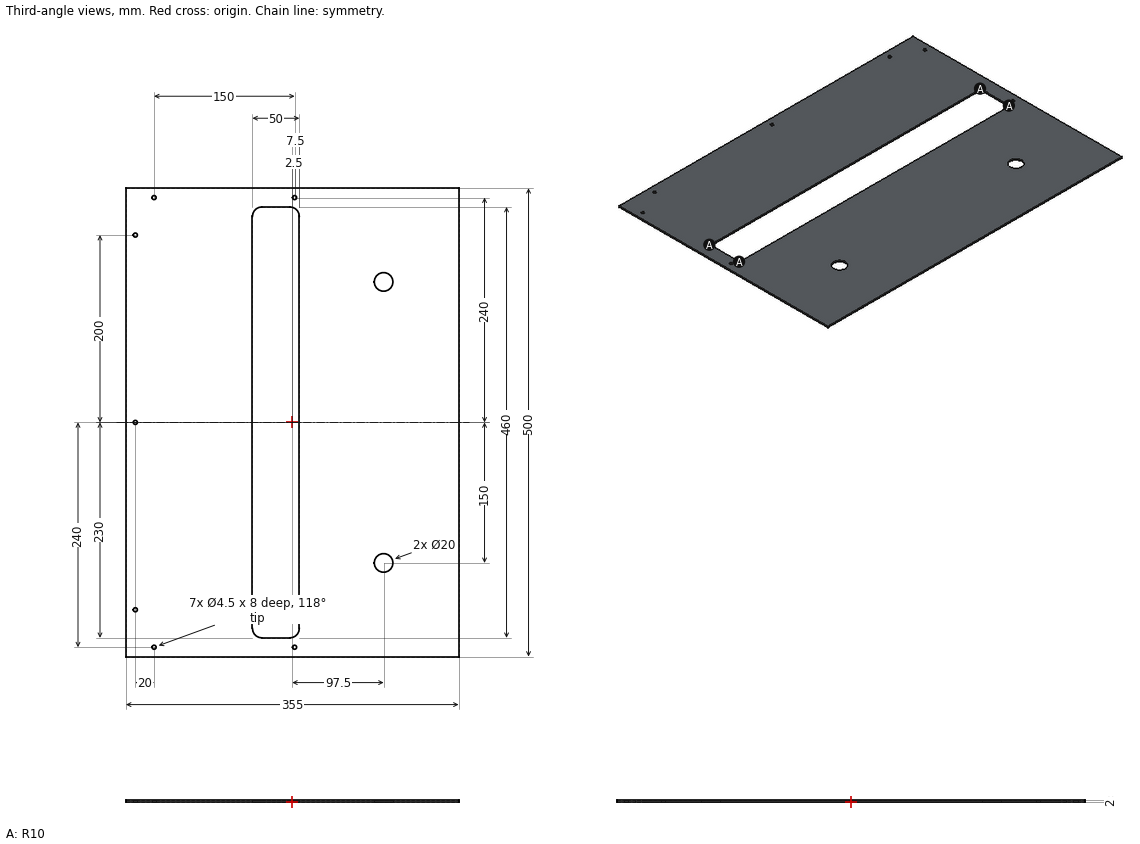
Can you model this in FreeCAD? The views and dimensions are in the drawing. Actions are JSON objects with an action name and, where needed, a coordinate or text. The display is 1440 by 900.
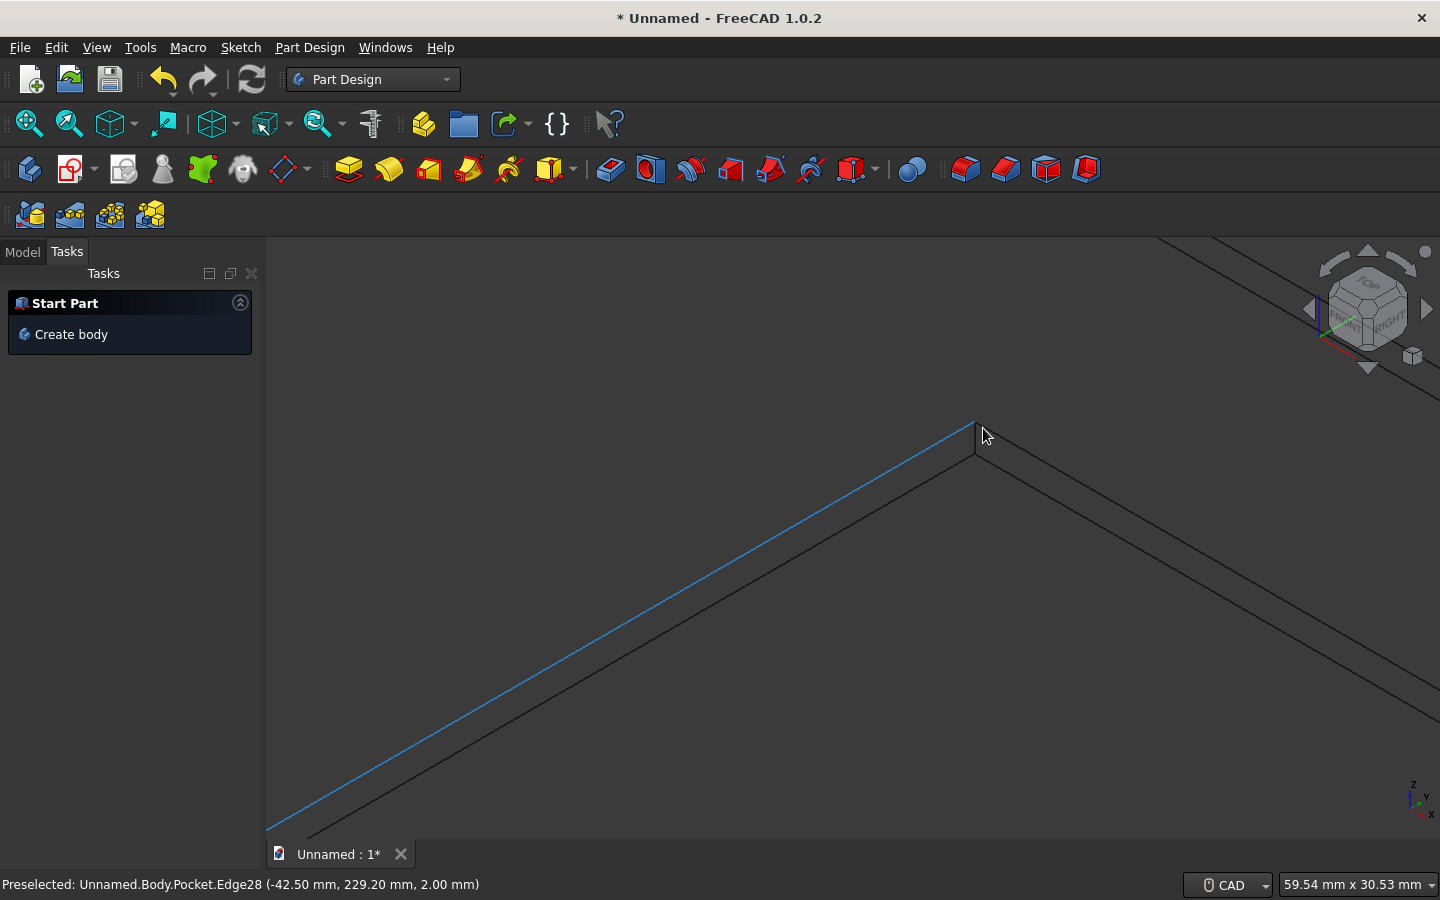
{"action": "left_click", "coordinate": [975, 437]}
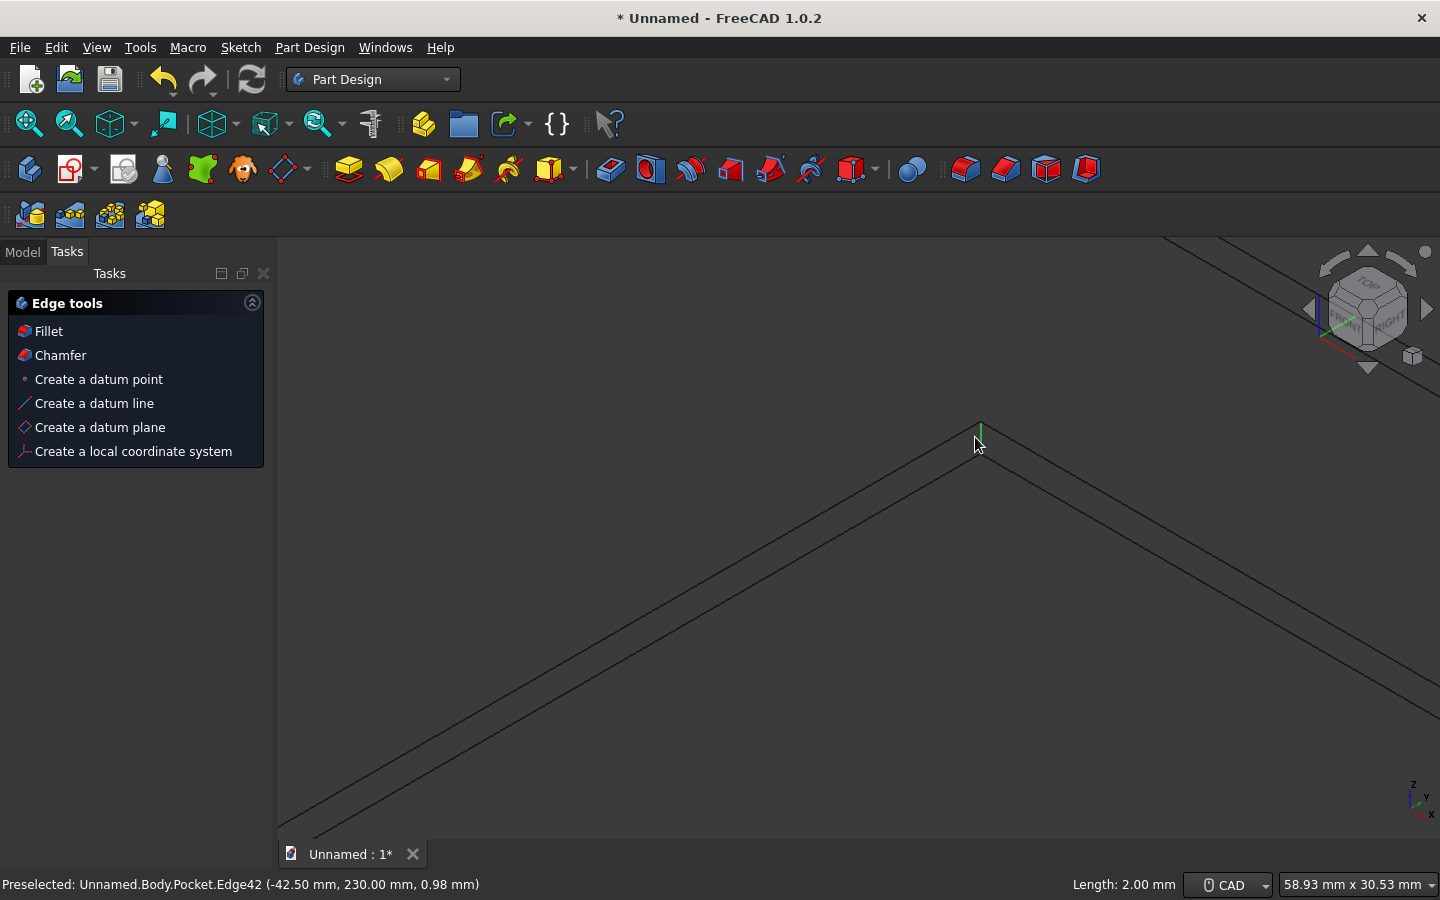
{"action": "left_click", "coordinate": [30, 124]}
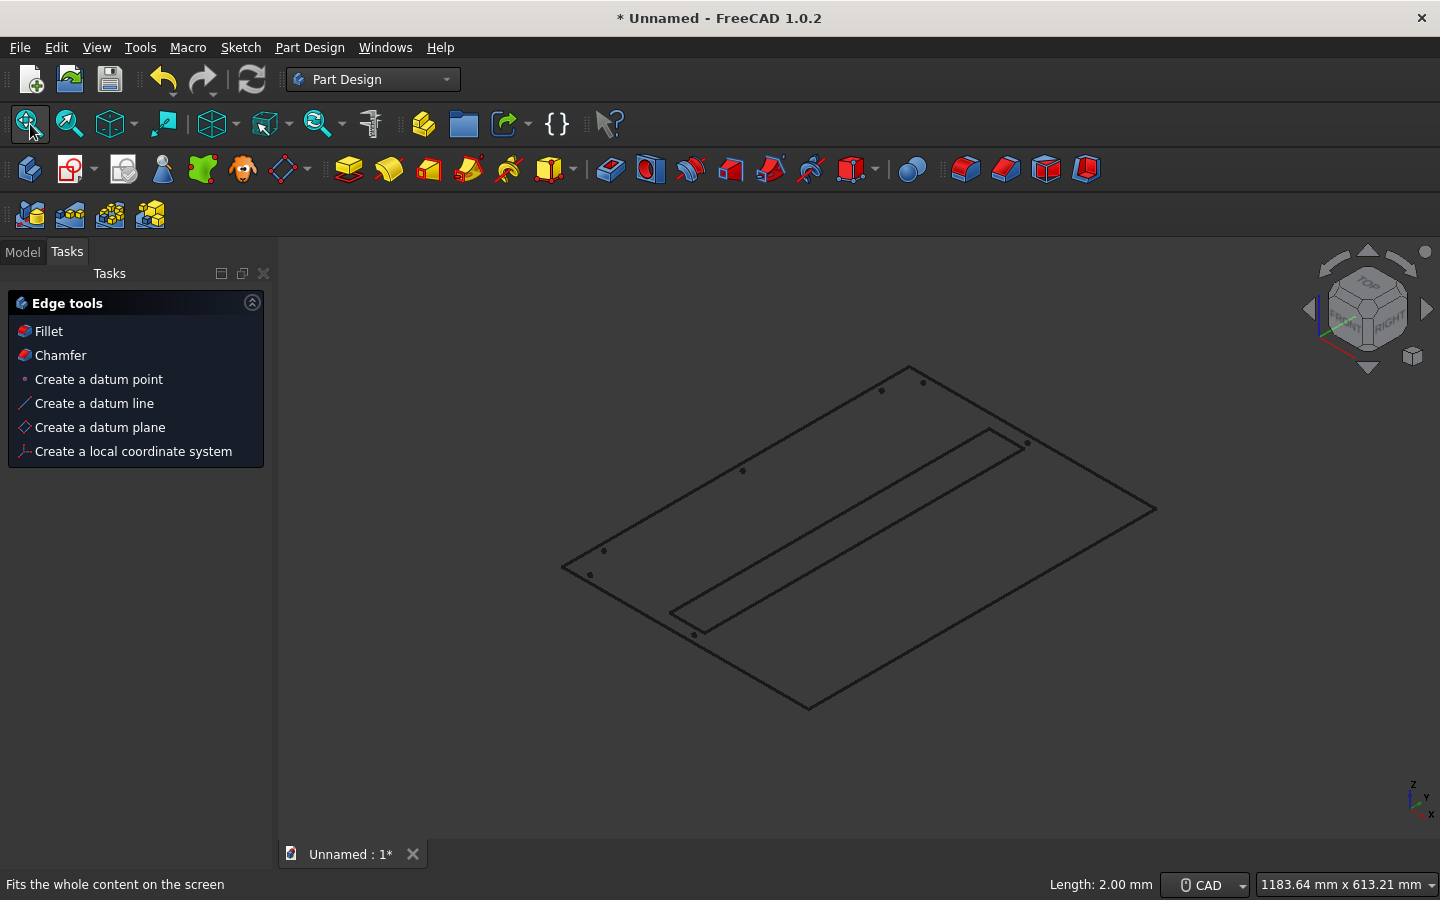
{"action": "key", "text": "2"}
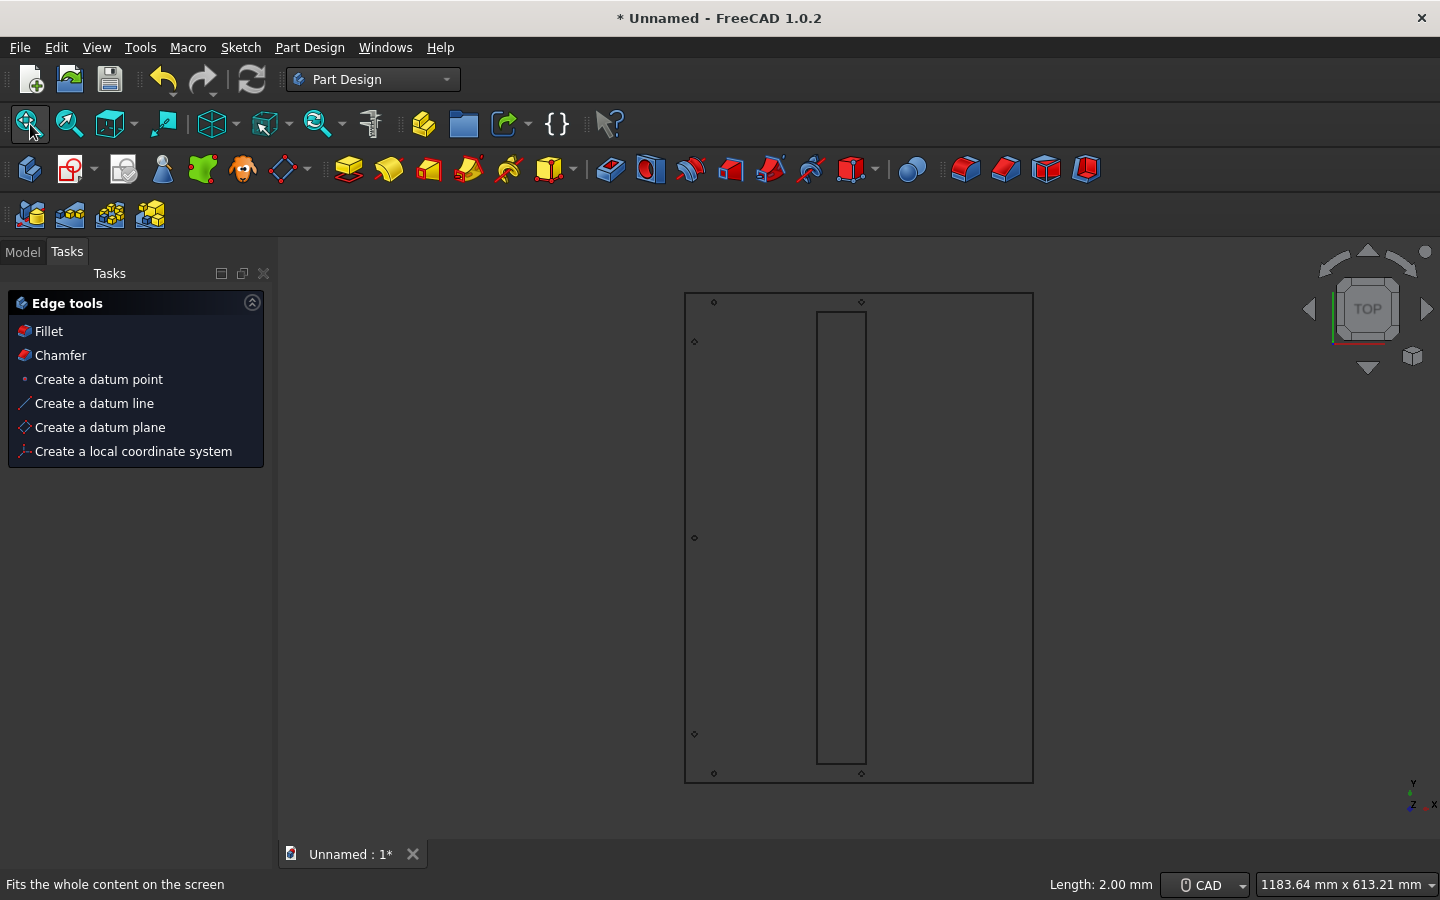
{"action": "scroll", "coordinate": [817, 763], "scroll_direction": "up", "scroll_amount": 15}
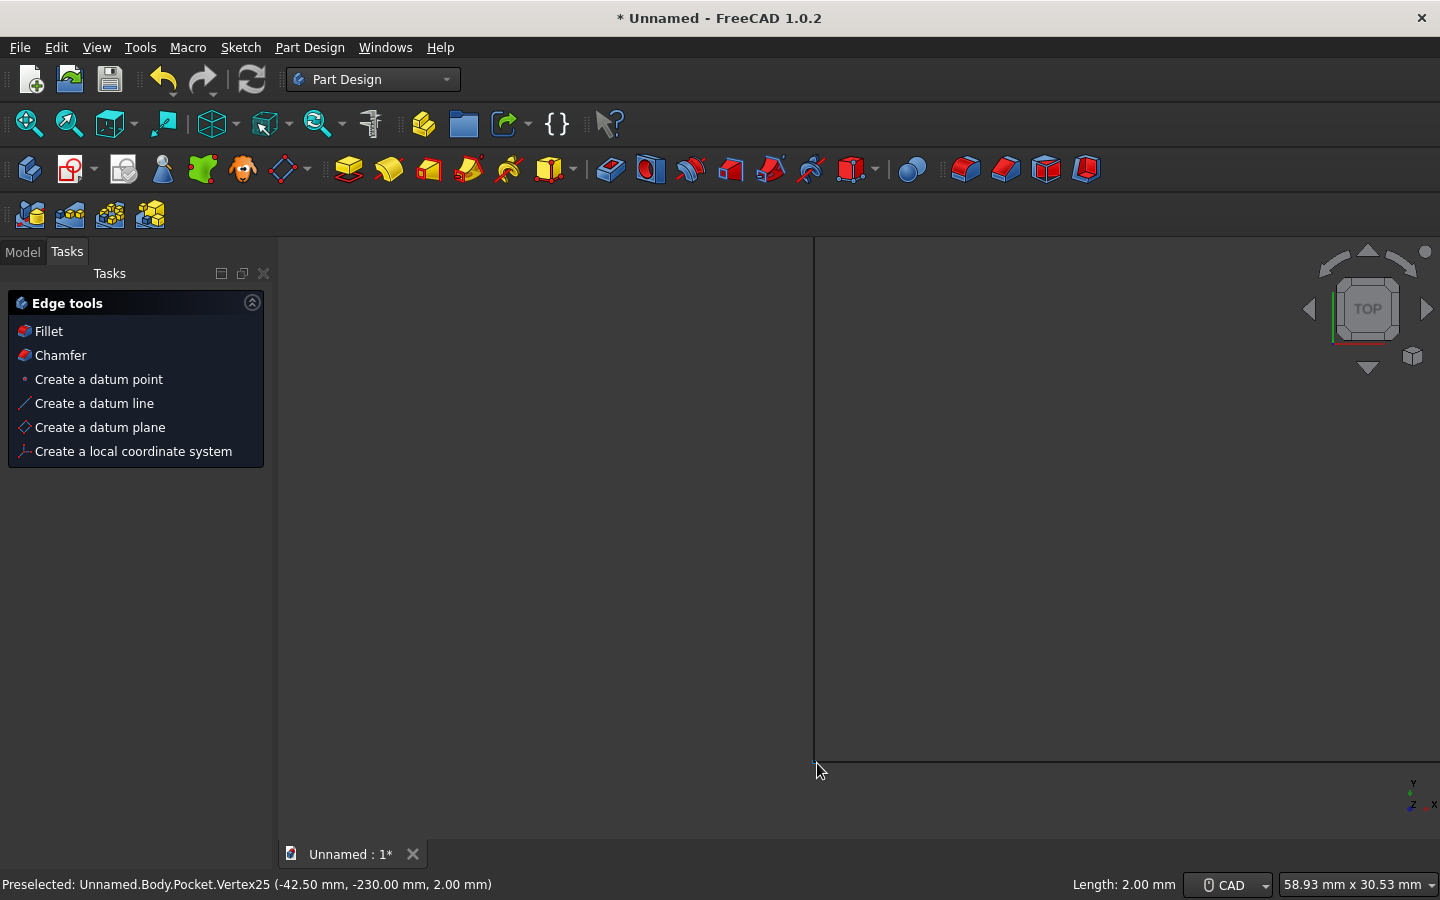
{"action": "left_click", "coordinate": [30, 124]}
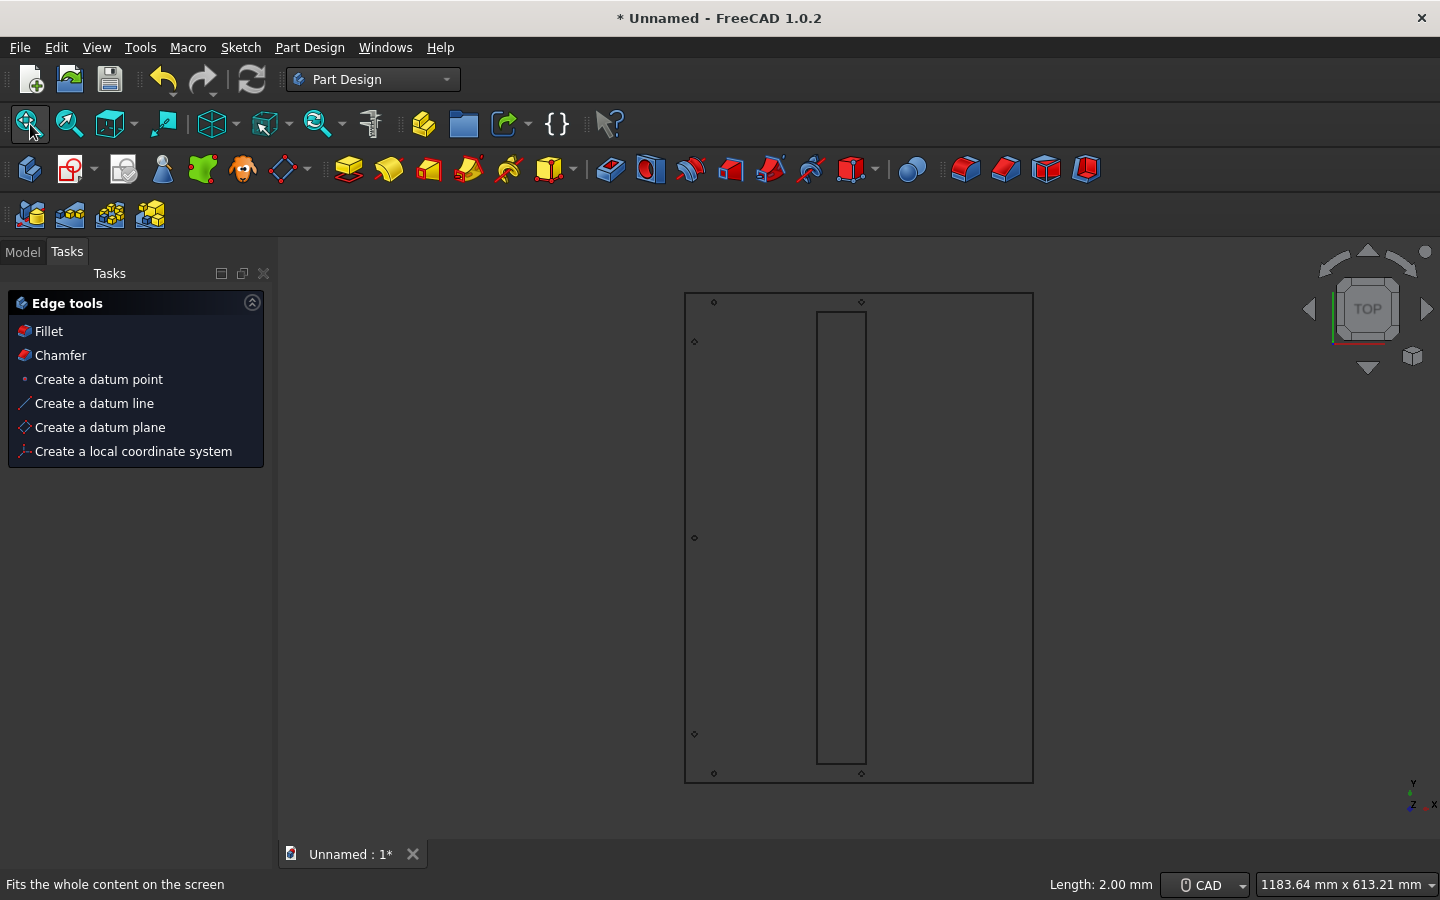
{"action": "key", "text": "1"}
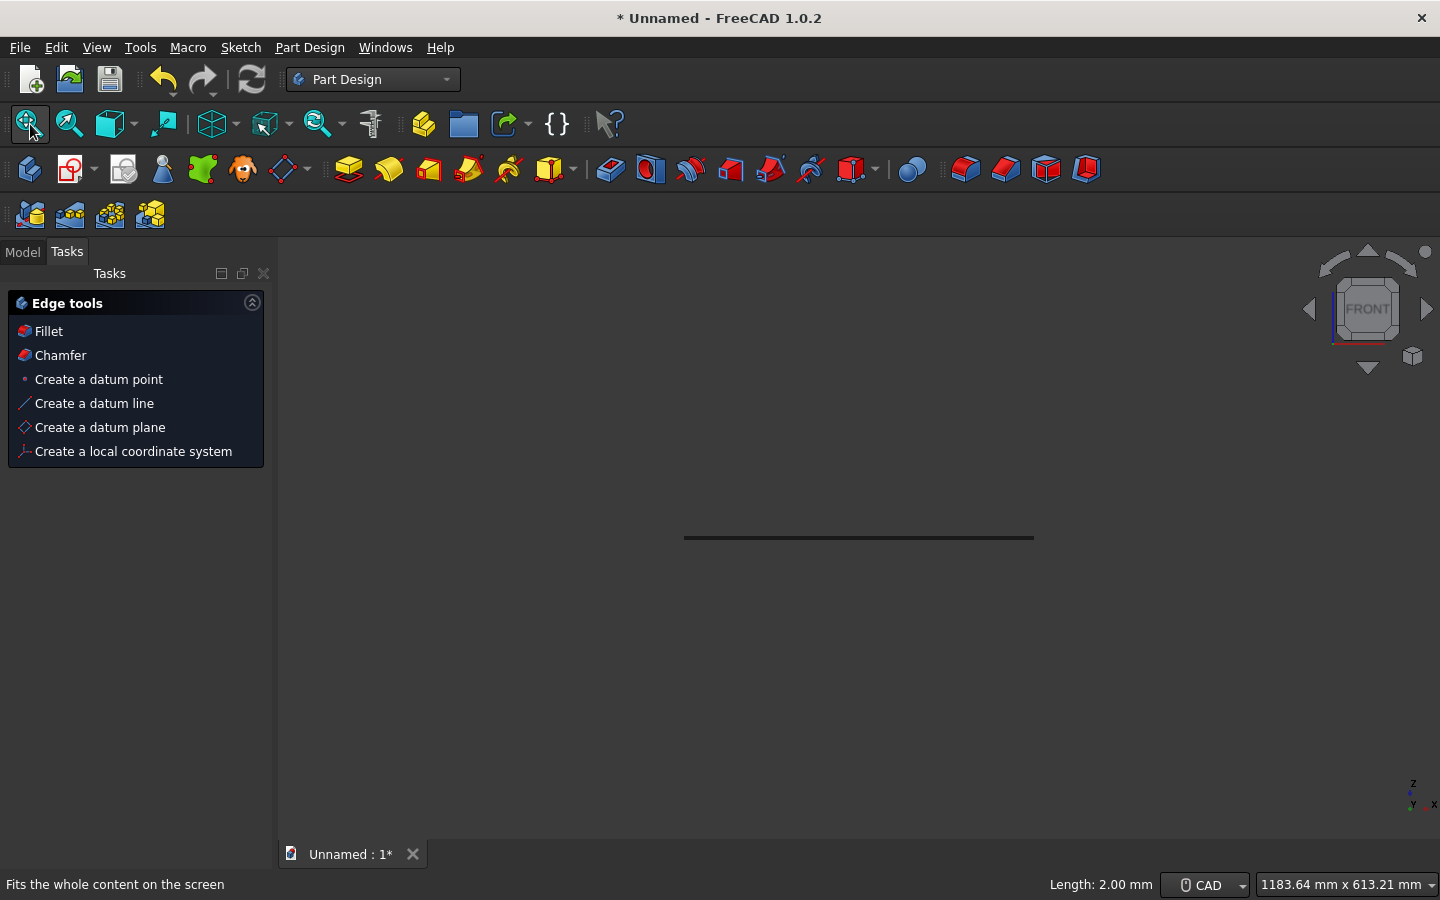
{"action": "left_click", "coordinate": [30, 124]}